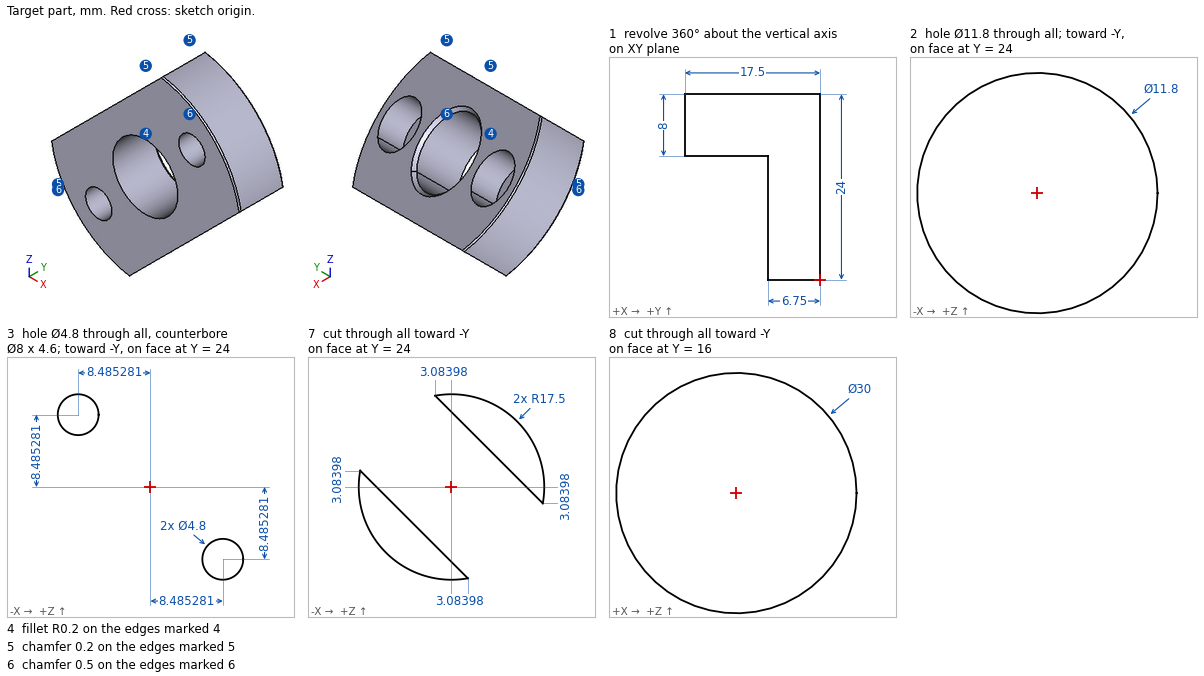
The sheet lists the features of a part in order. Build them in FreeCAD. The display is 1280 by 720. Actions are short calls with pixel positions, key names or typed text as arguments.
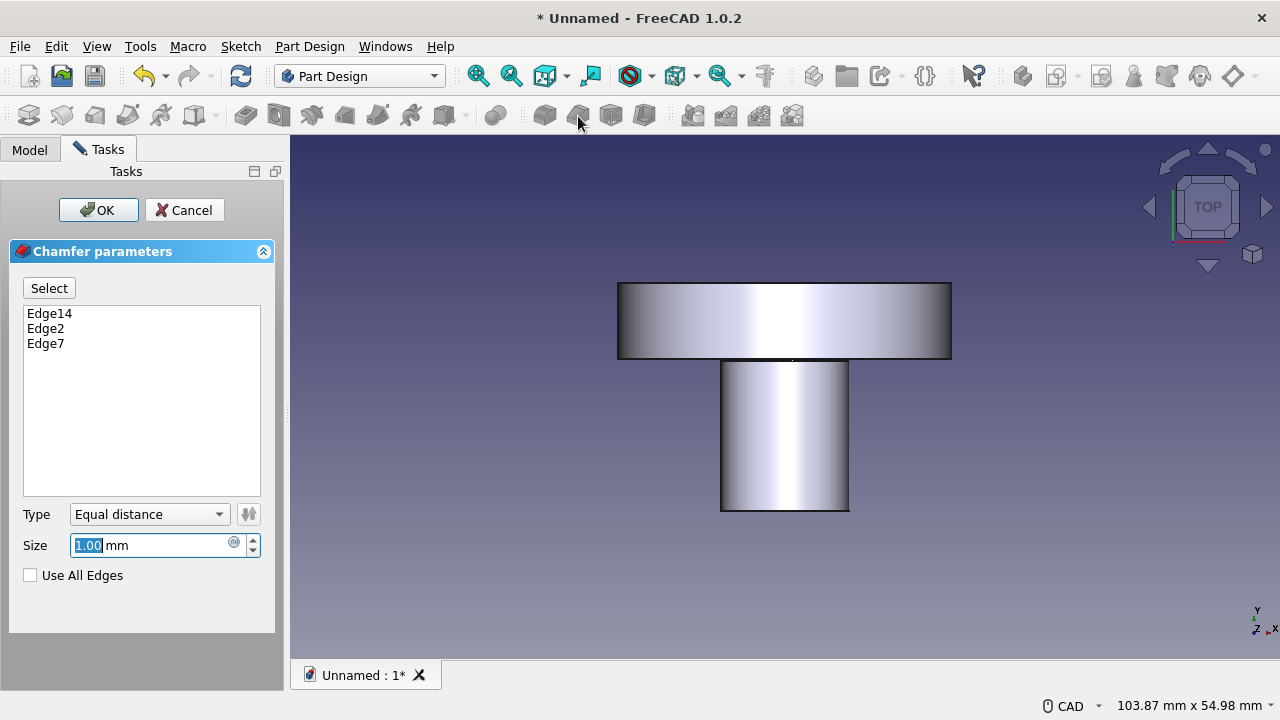
text(0.2)
key(Tab)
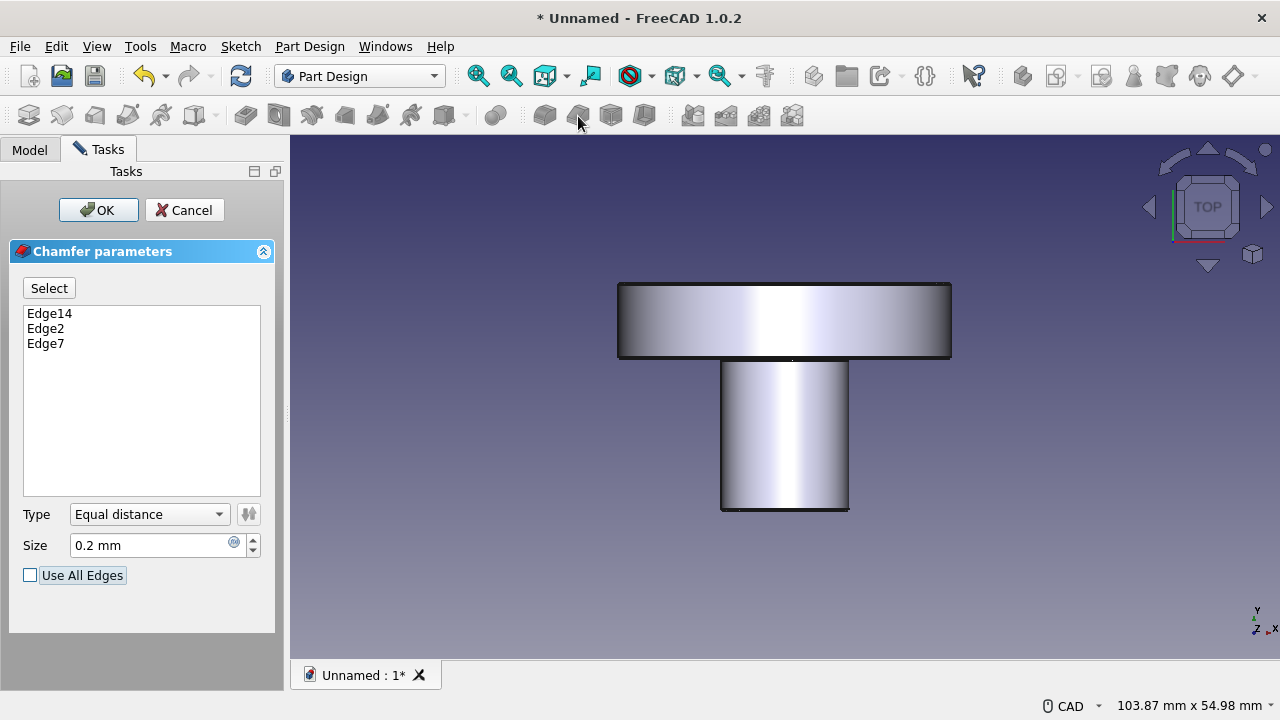
click(99, 210)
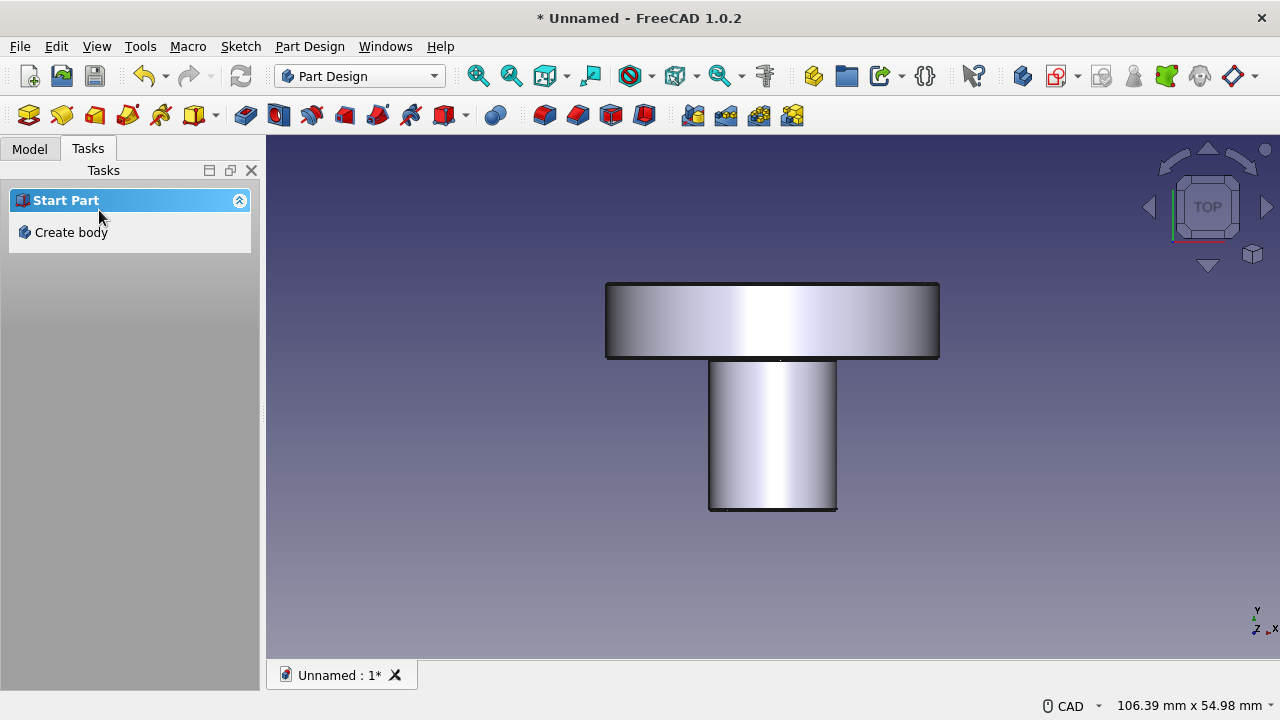
click(479, 76)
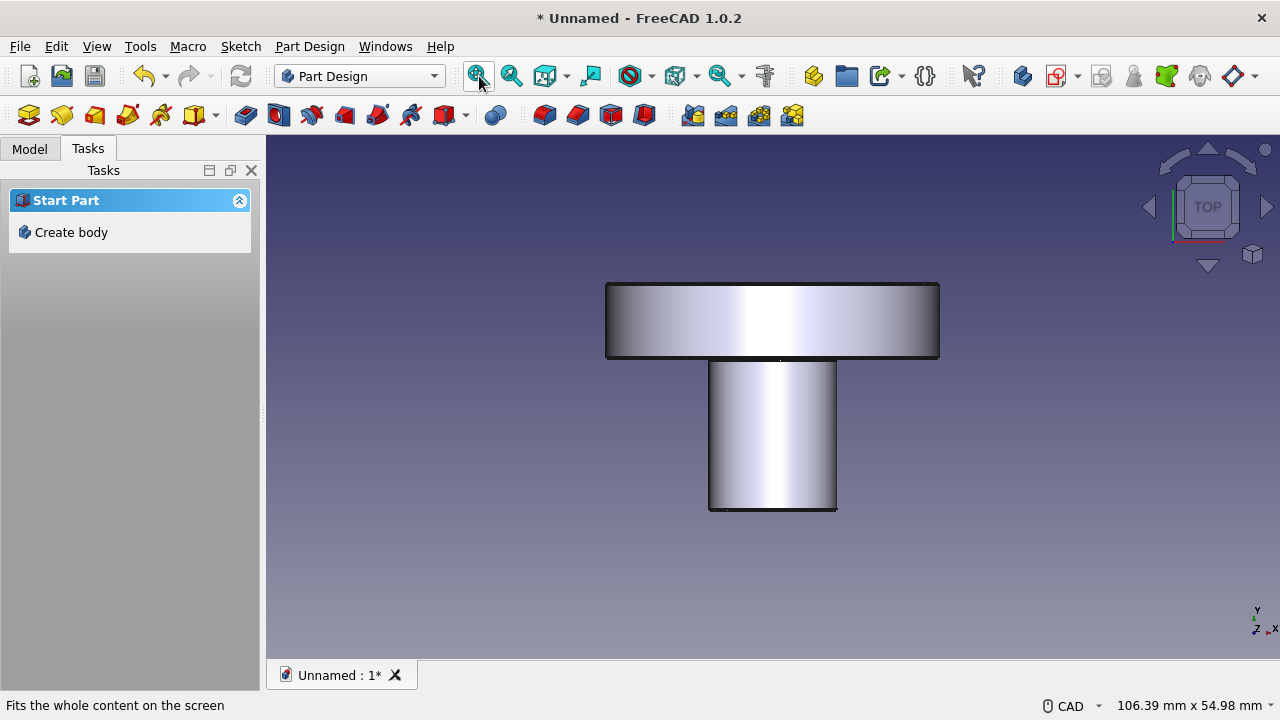
key(0)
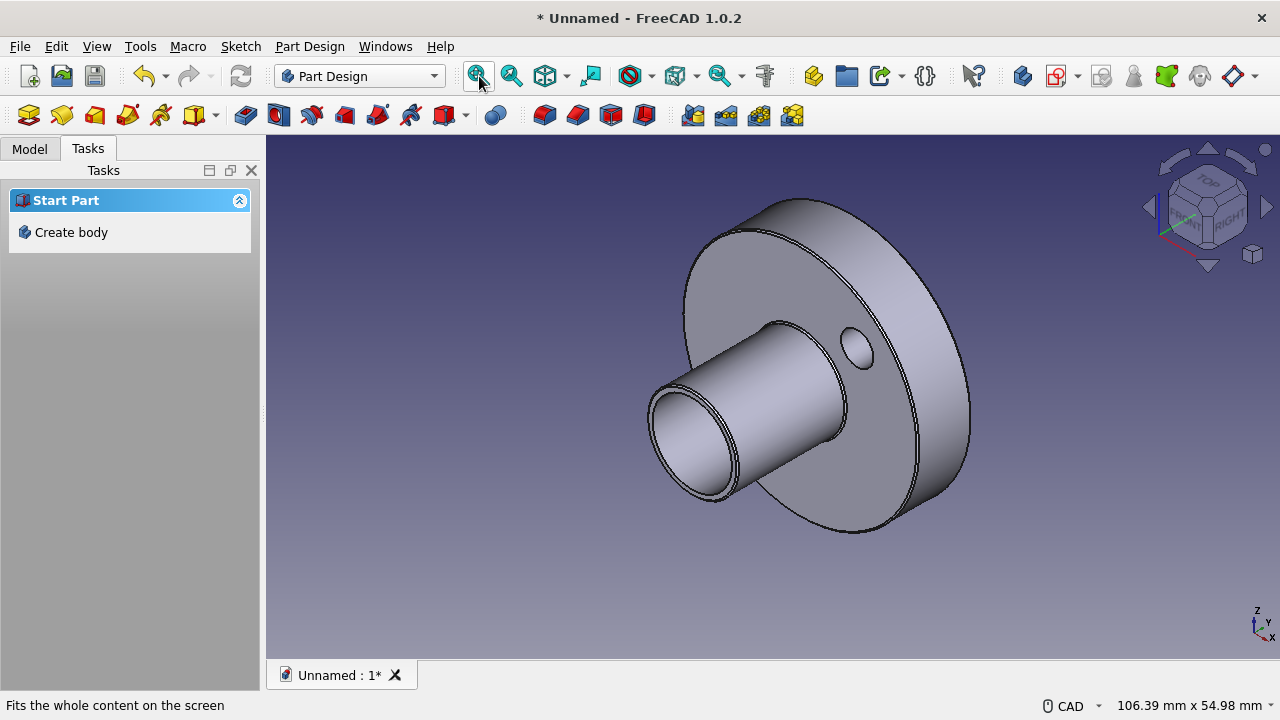
click(652, 420)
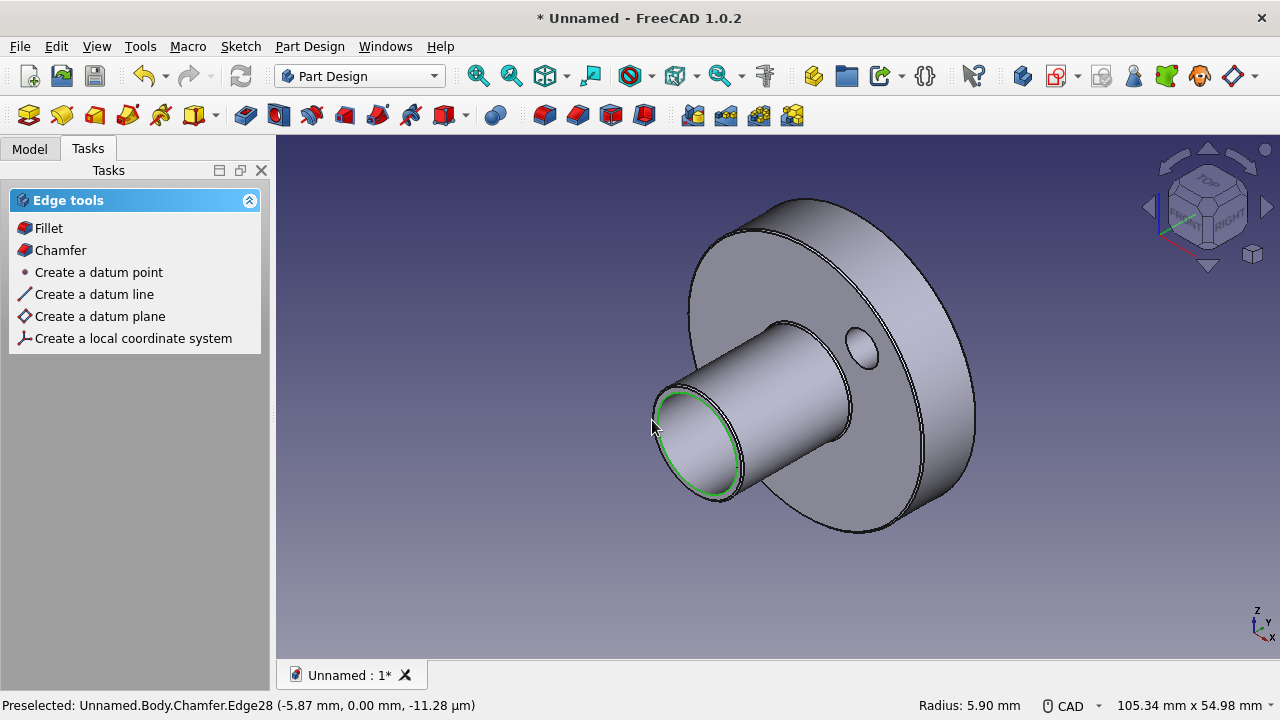
key(2)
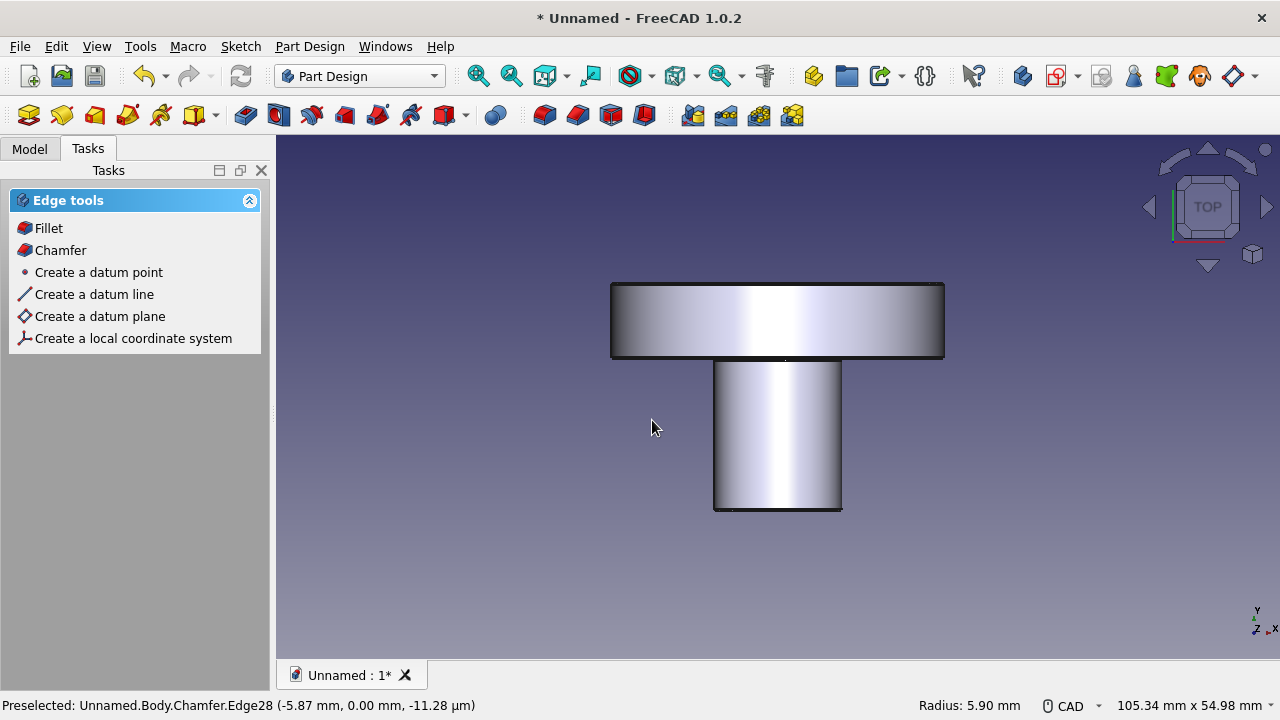
click(479, 76)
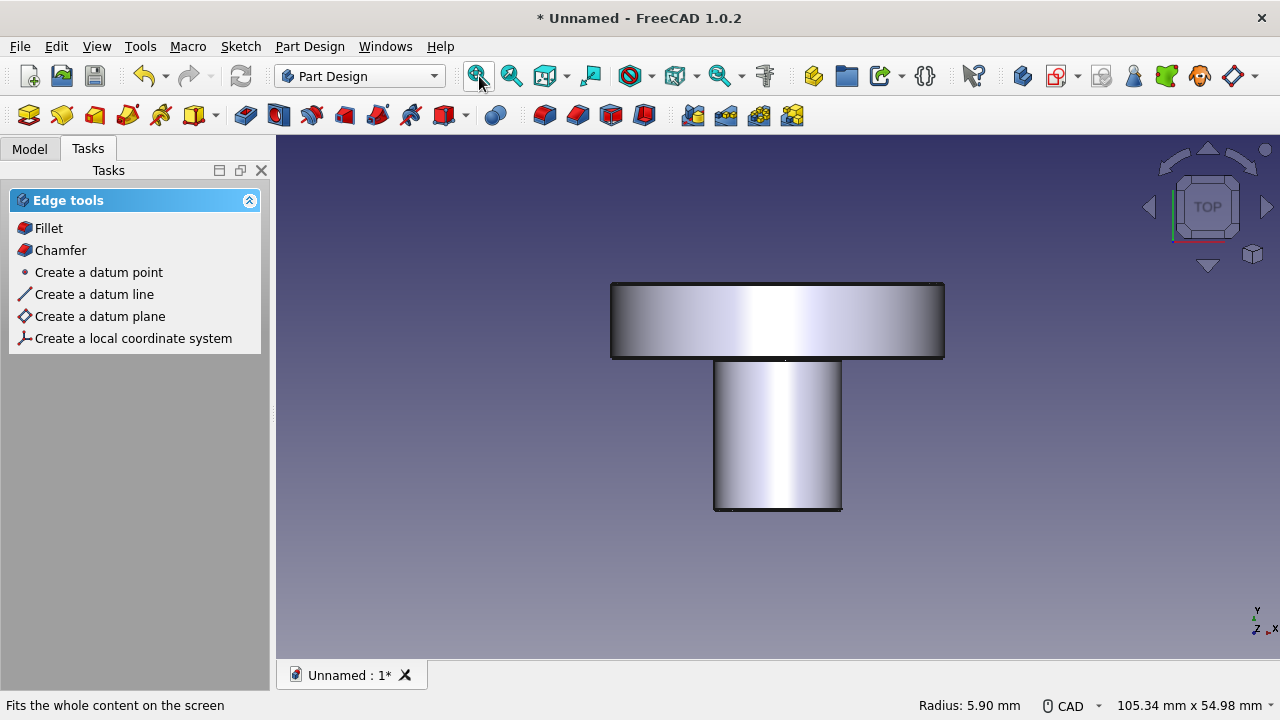
key(1)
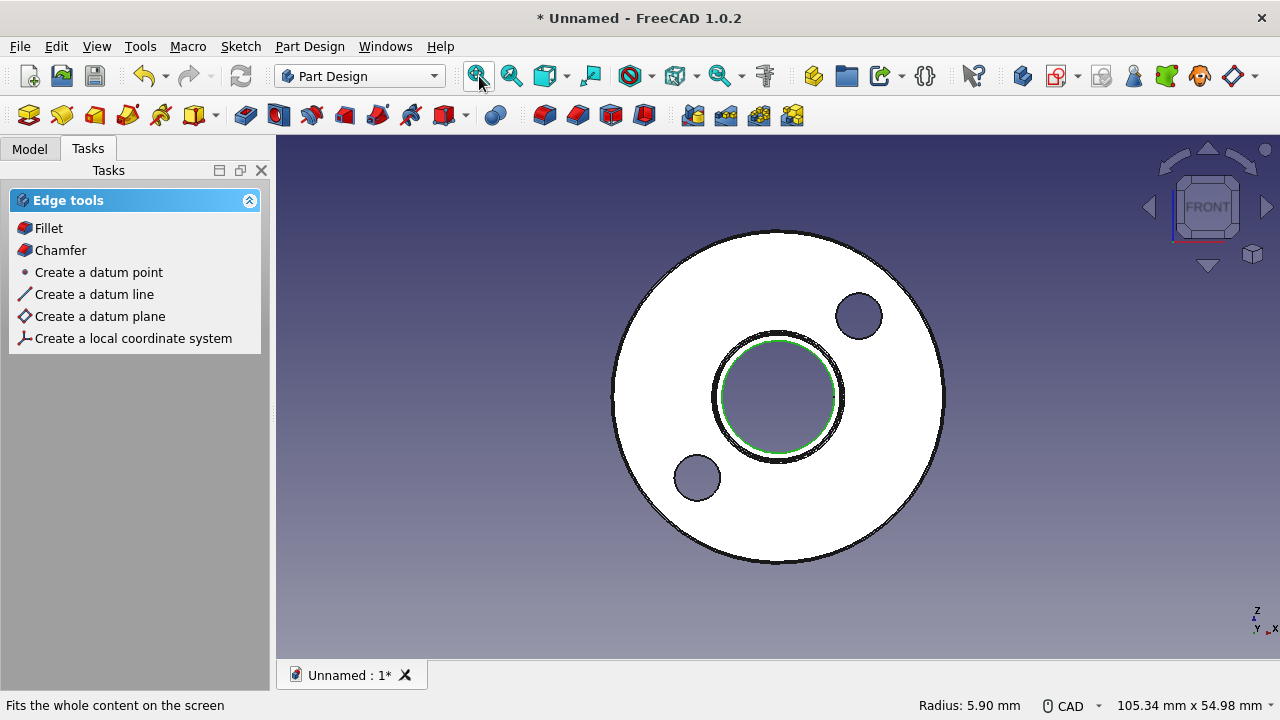
key(3)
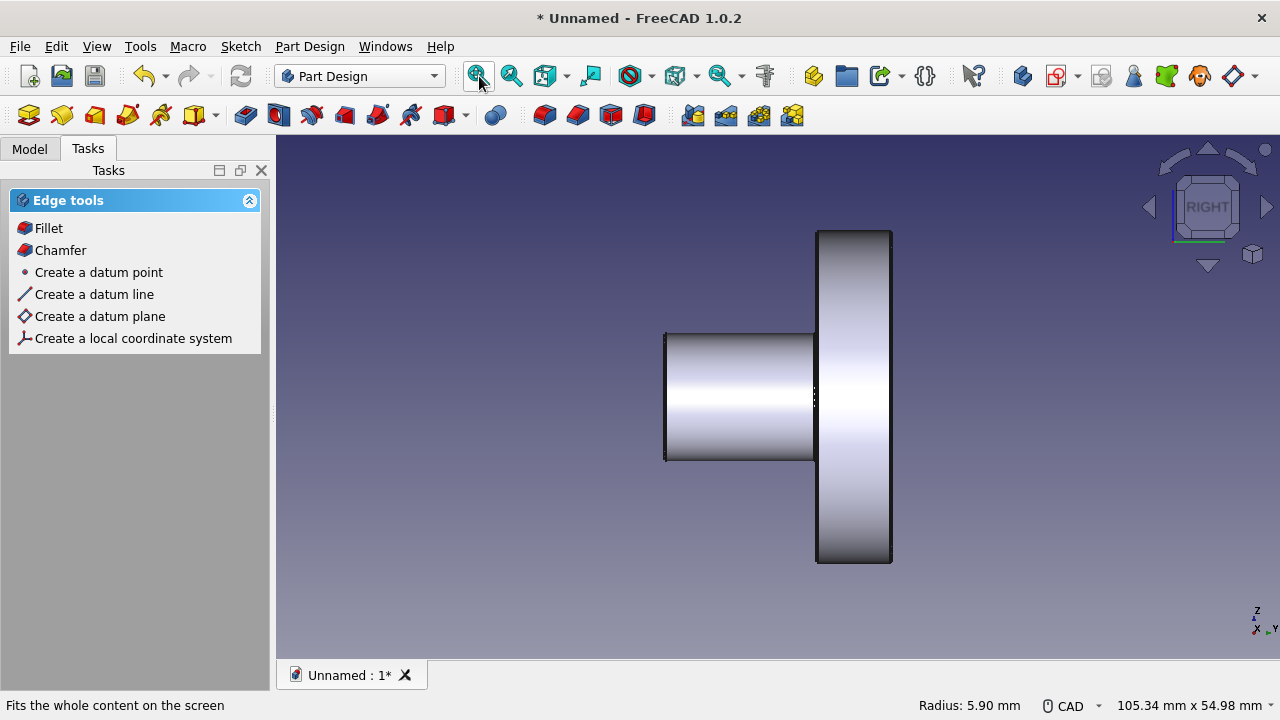
key(5)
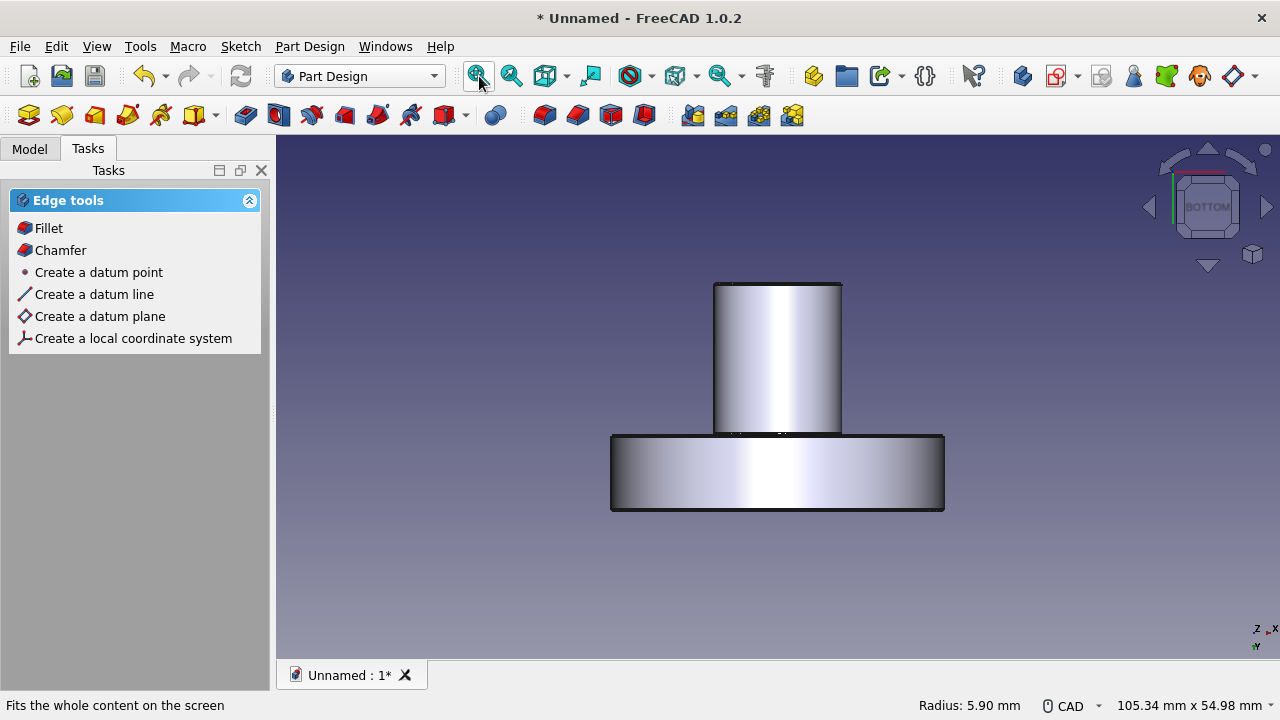
click(479, 76)